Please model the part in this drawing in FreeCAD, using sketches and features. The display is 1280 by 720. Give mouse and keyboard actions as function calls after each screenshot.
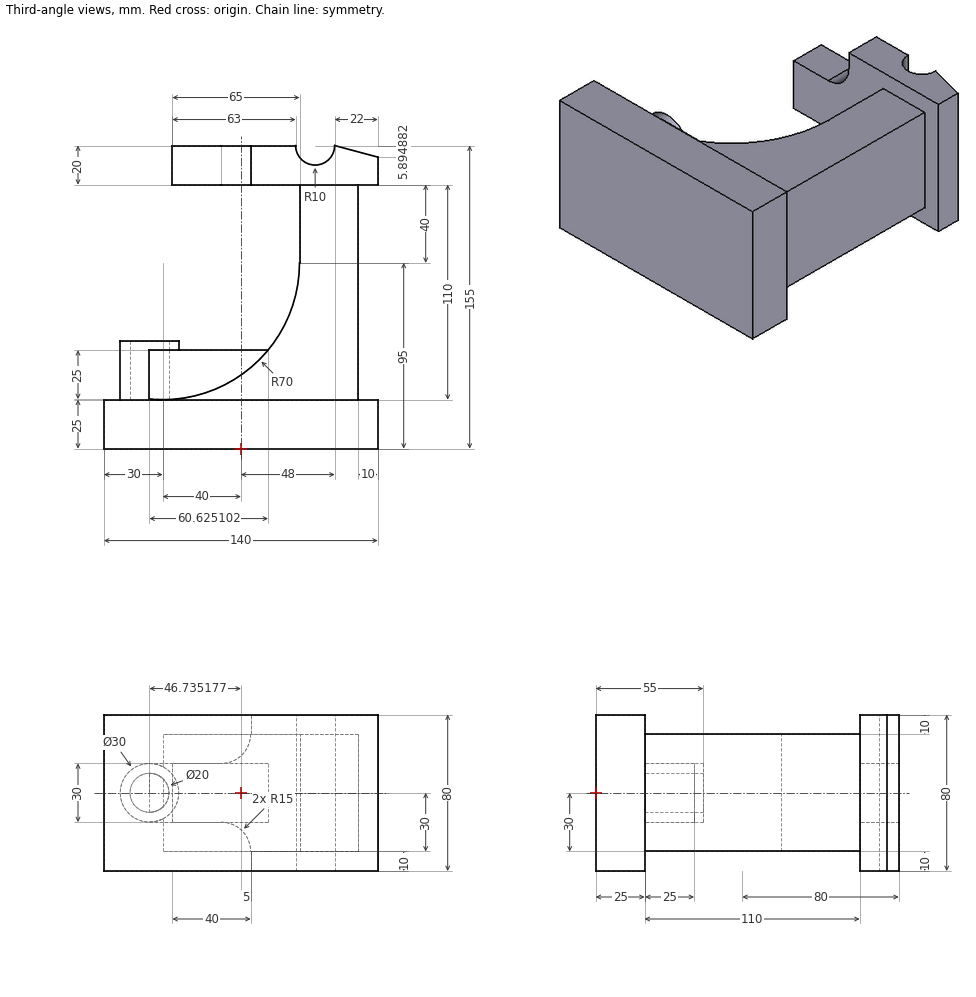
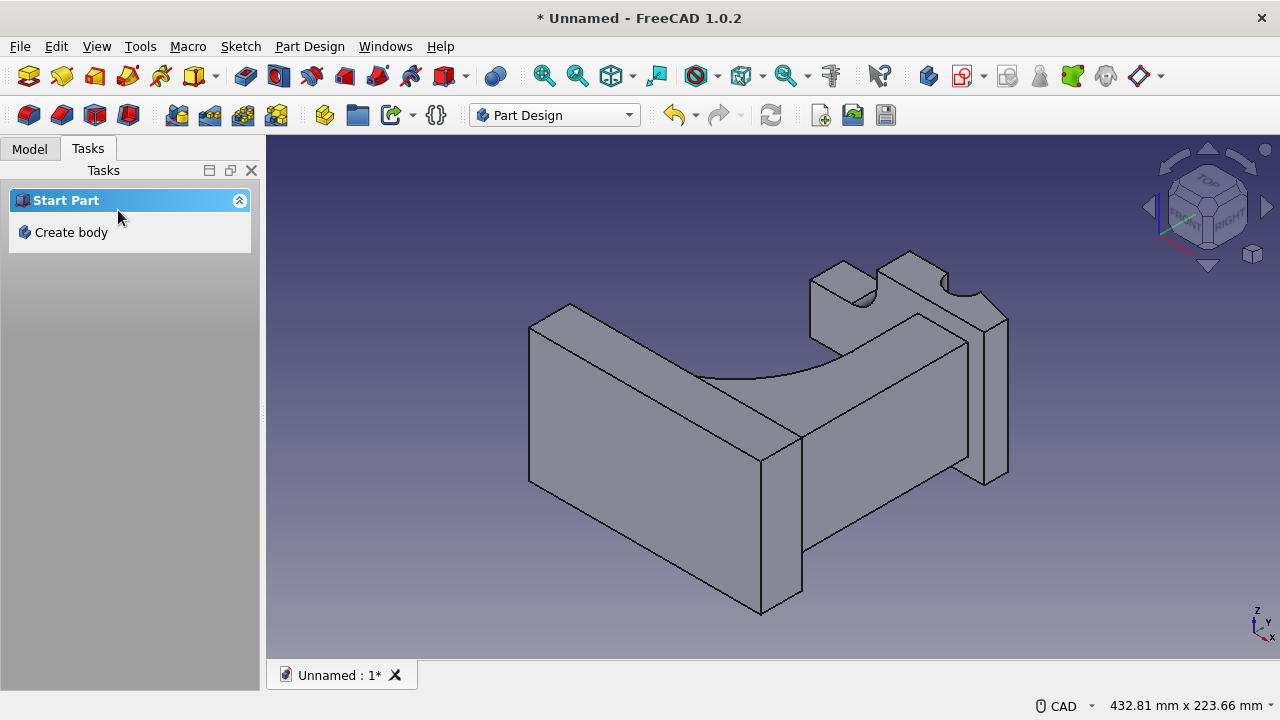
click(678, 489)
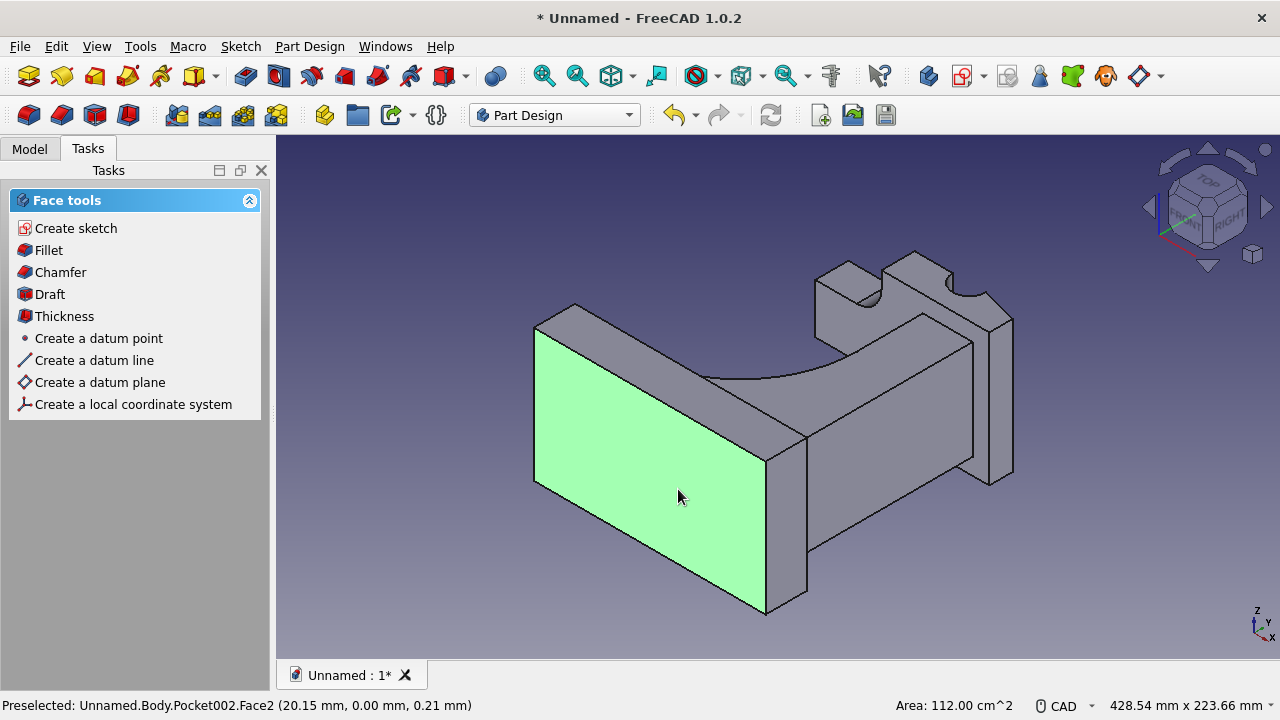
click(962, 76)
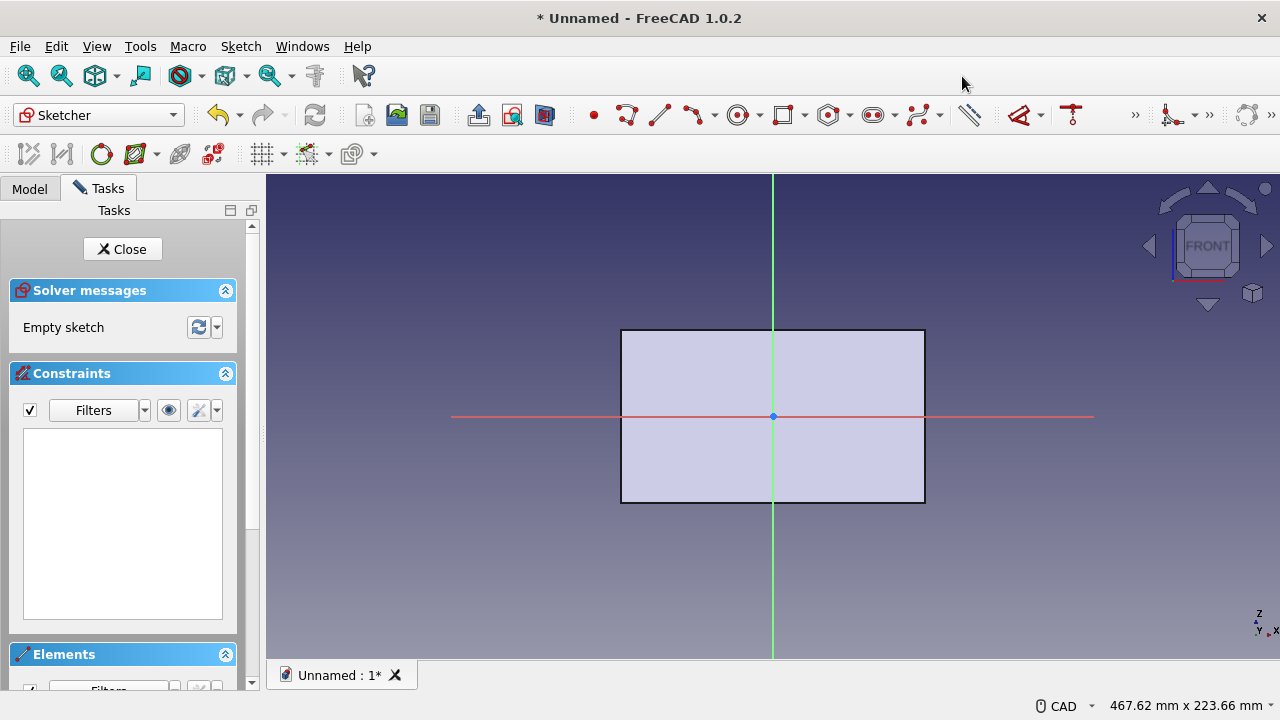
scroll(707, 417, up, 7)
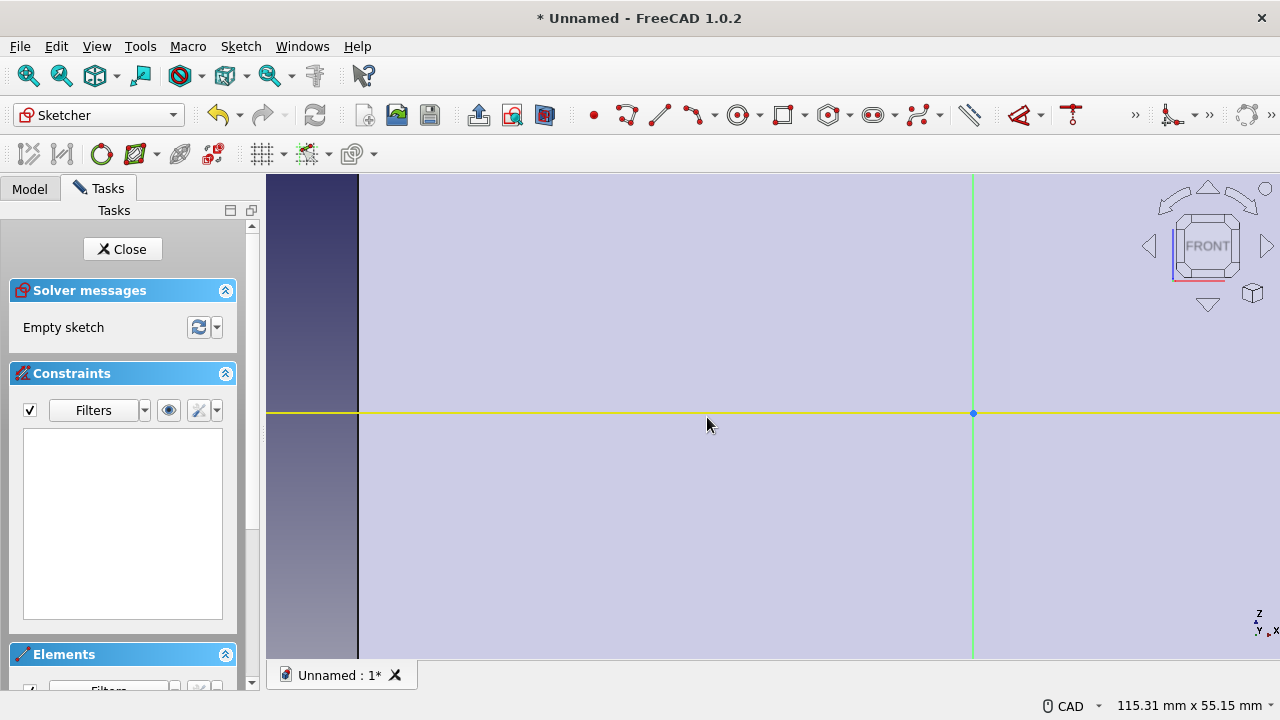
click(738, 116)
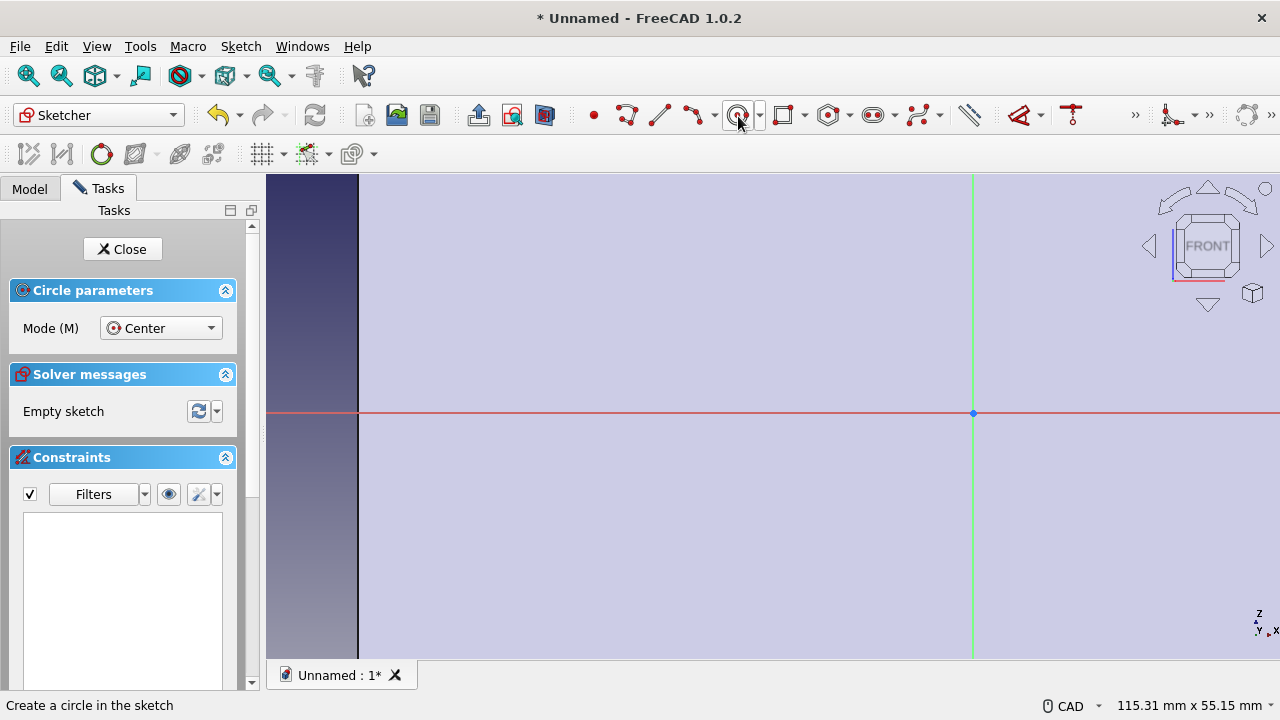
click(562, 413)
move(656, 320)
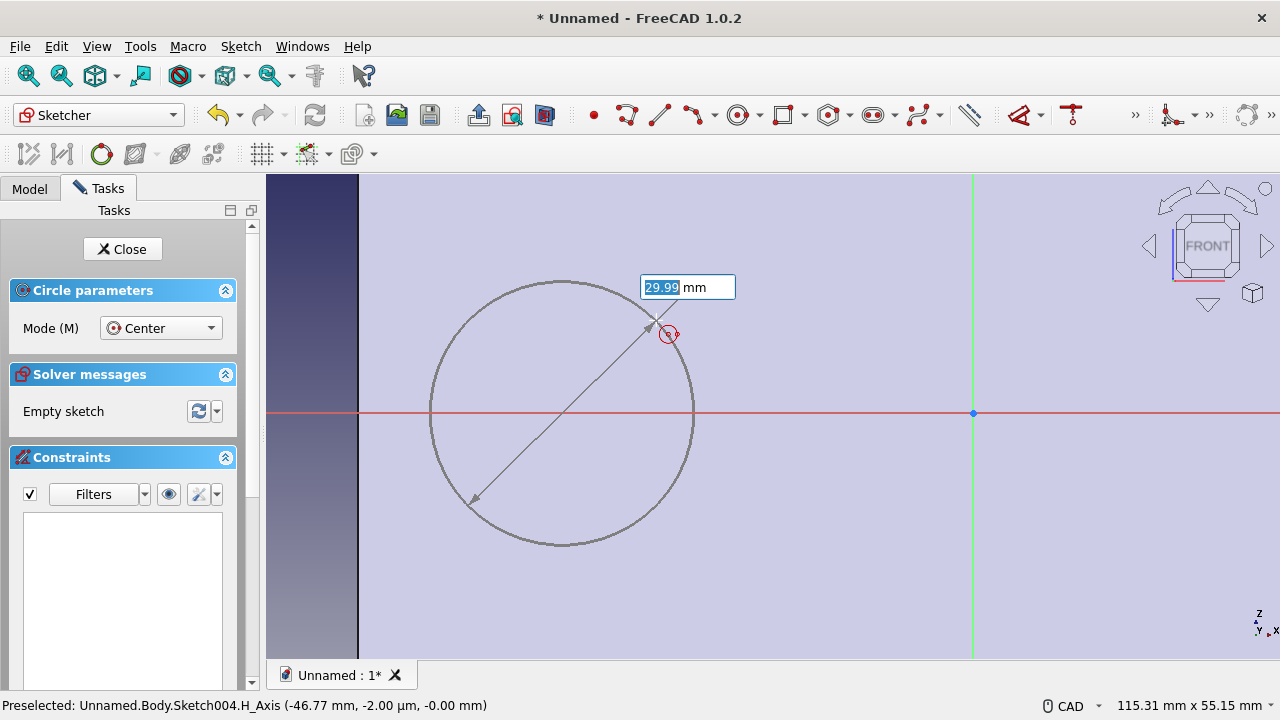
text(30)
key(Return)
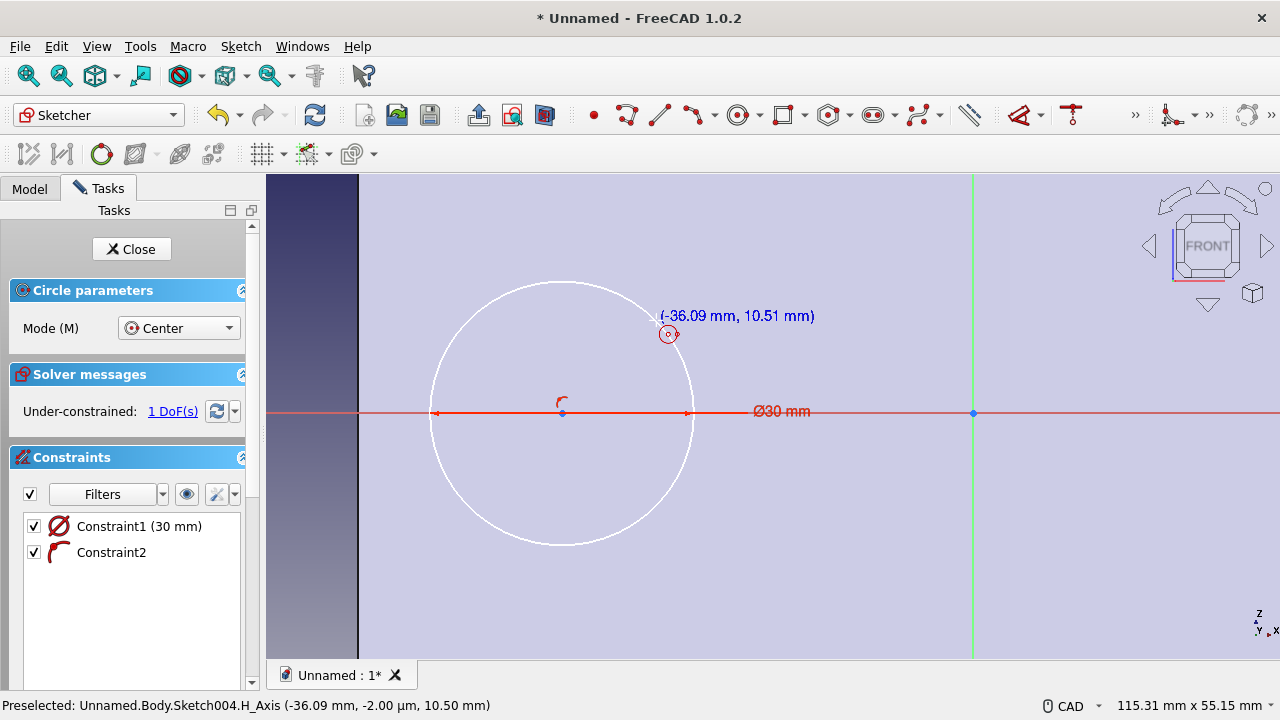
click(562, 413)
move(625, 351)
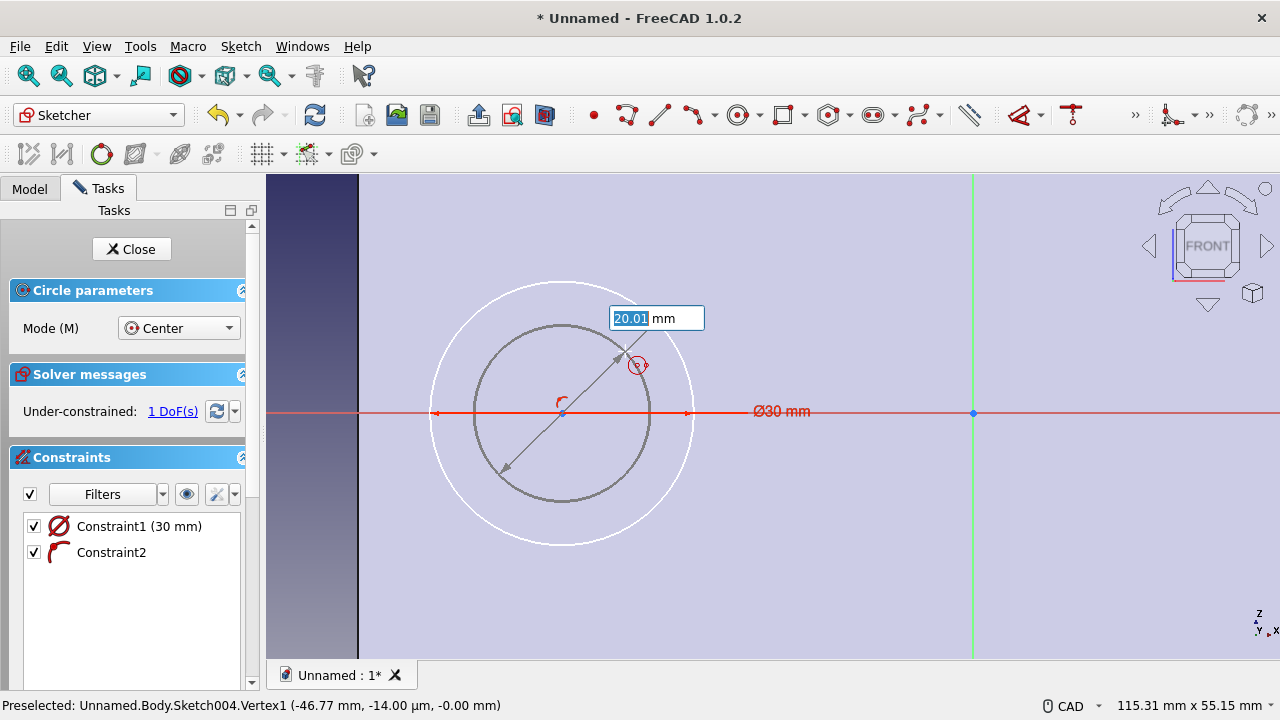
text(20)
key(Return)
key(Escape)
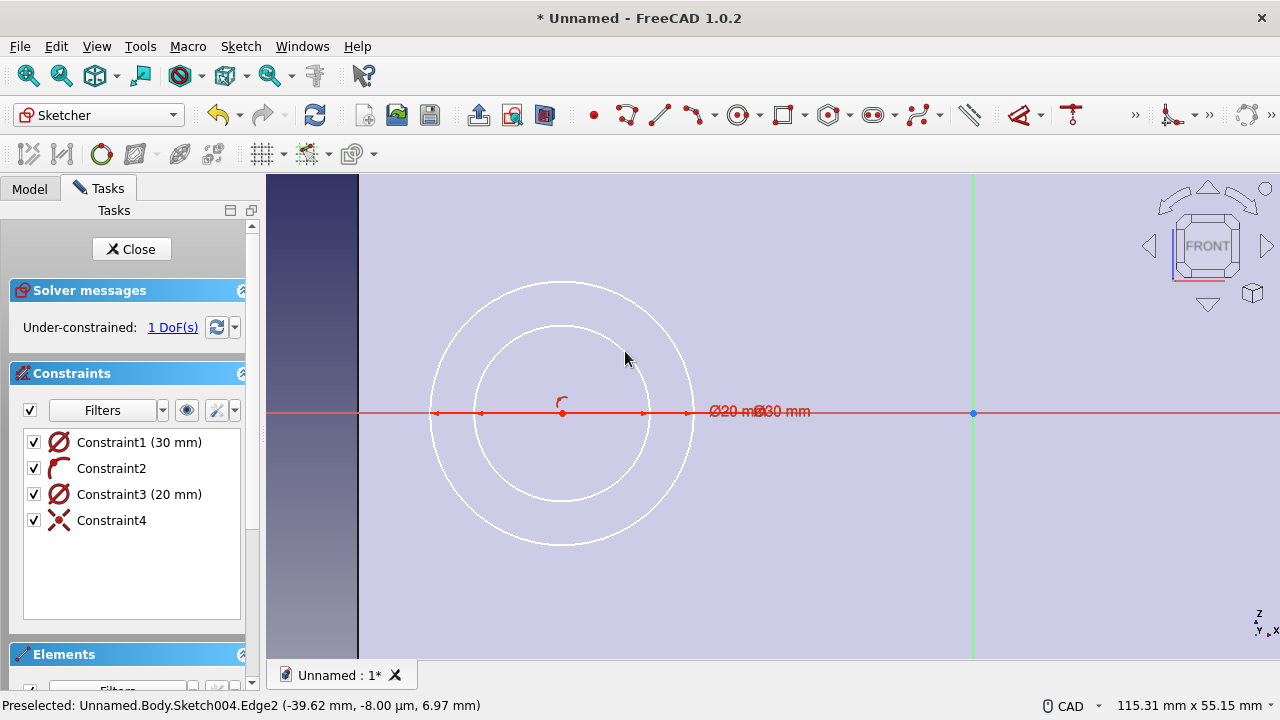
click(1018, 116)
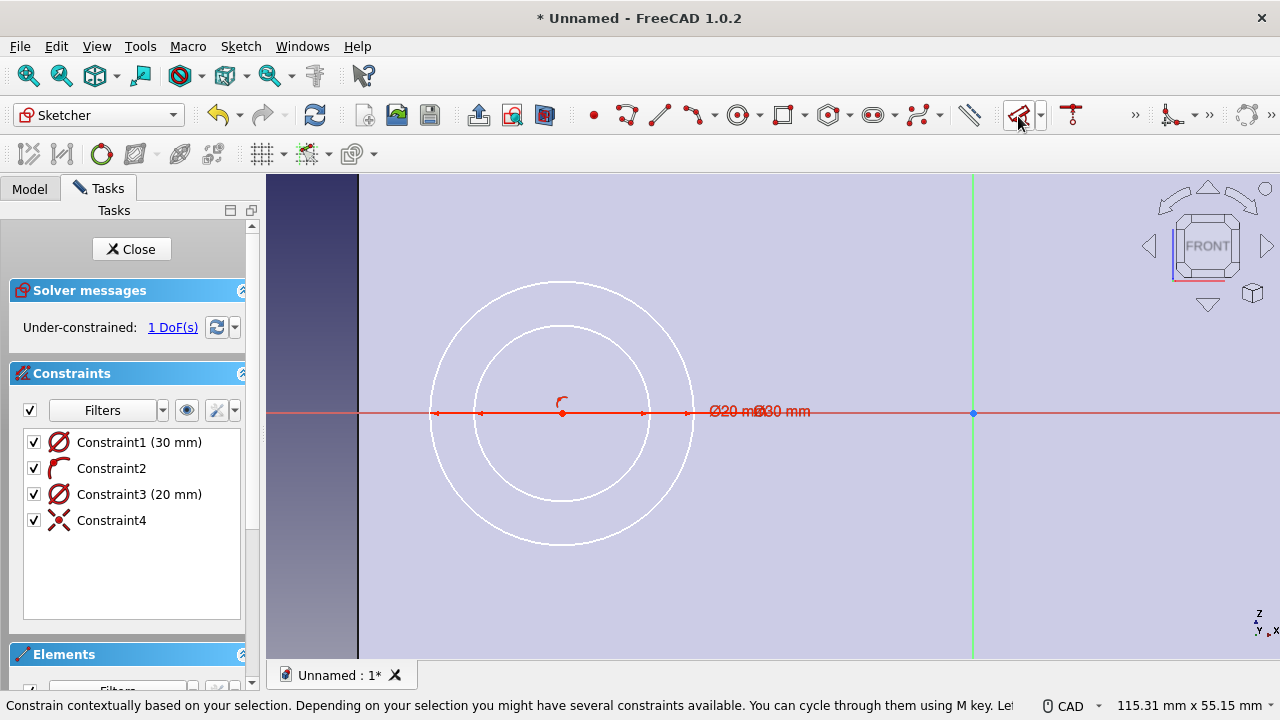
click(562, 413)
click(768, 447)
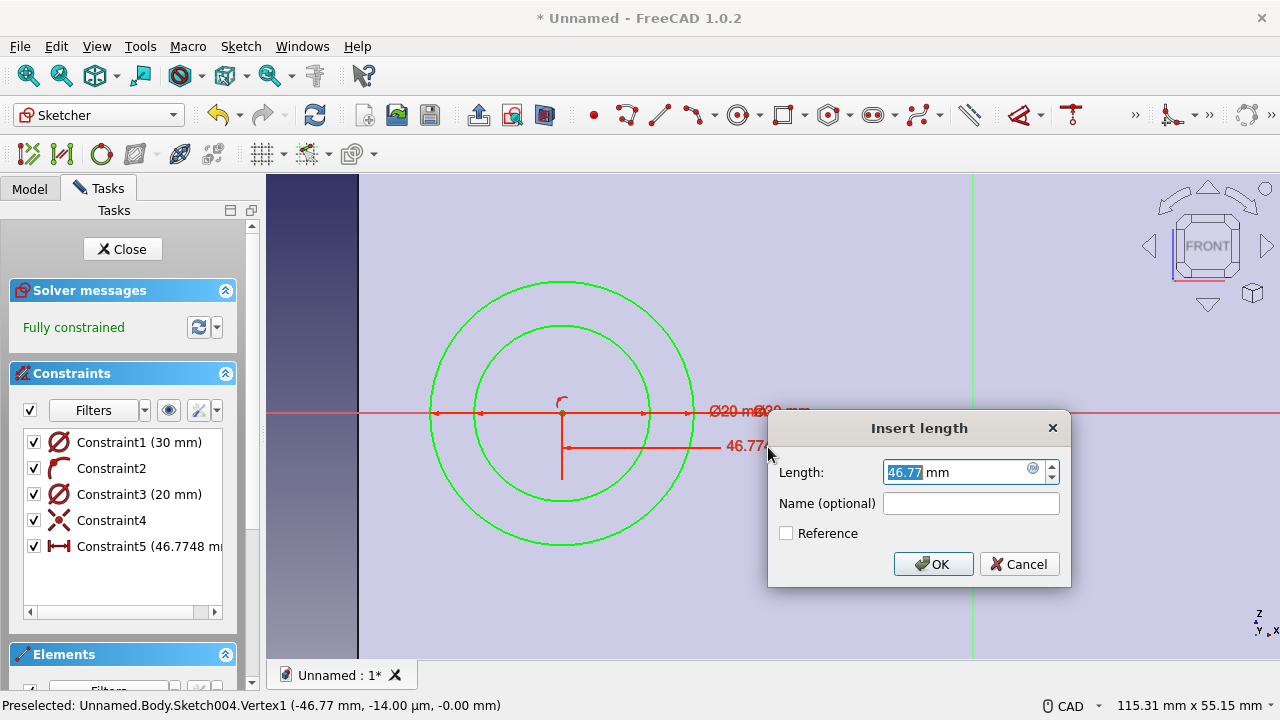
text(46.735177)
key(Return)
key(Escape)